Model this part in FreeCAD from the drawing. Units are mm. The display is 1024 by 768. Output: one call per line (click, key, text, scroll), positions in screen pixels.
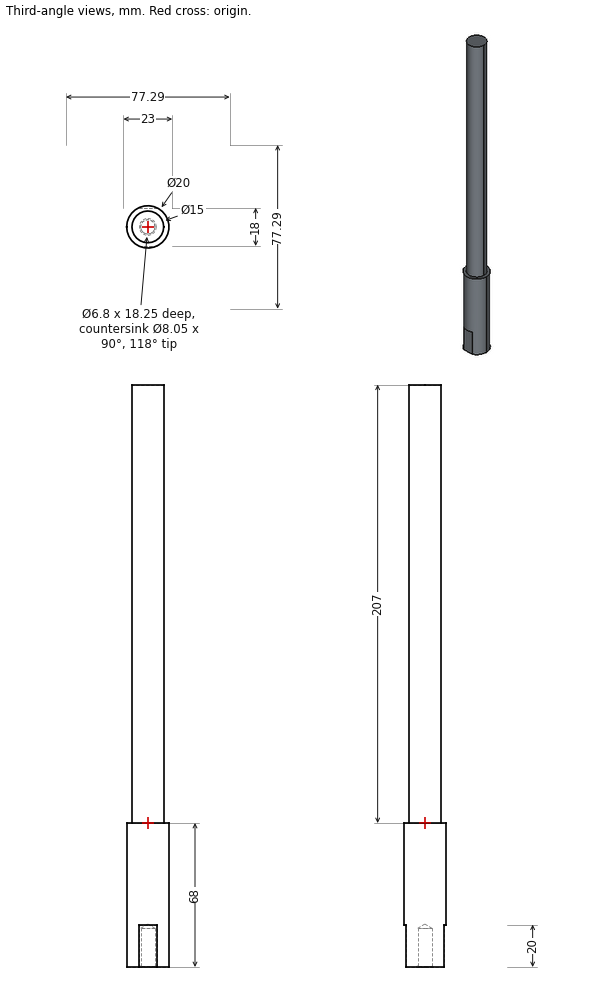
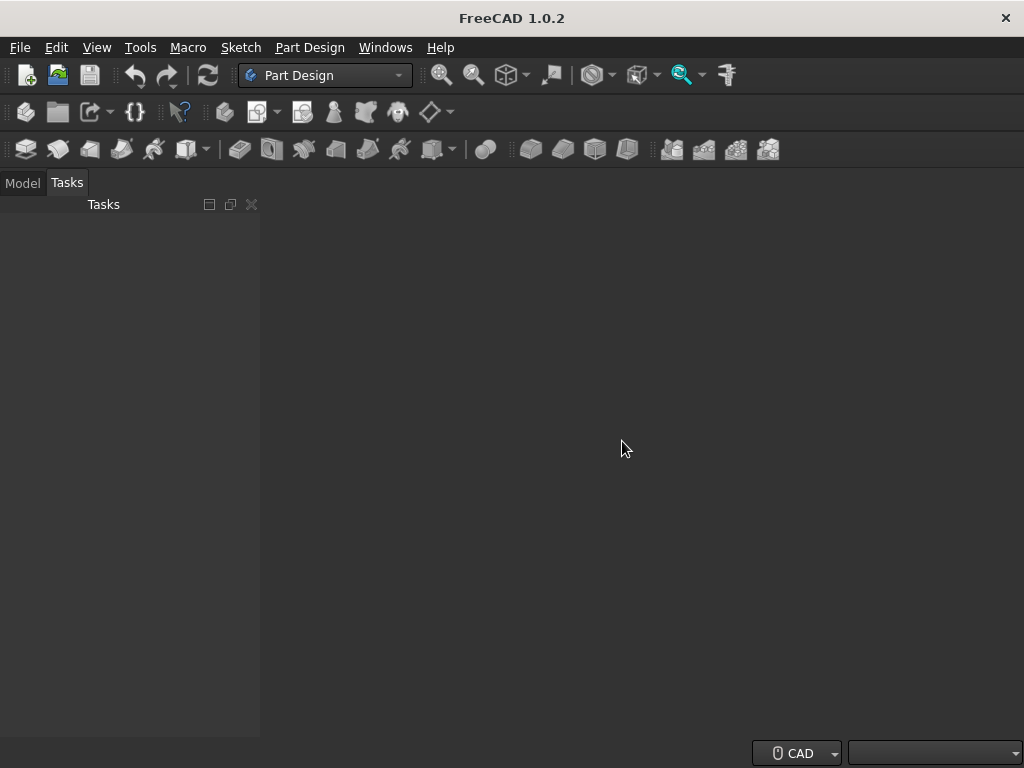
click(26, 76)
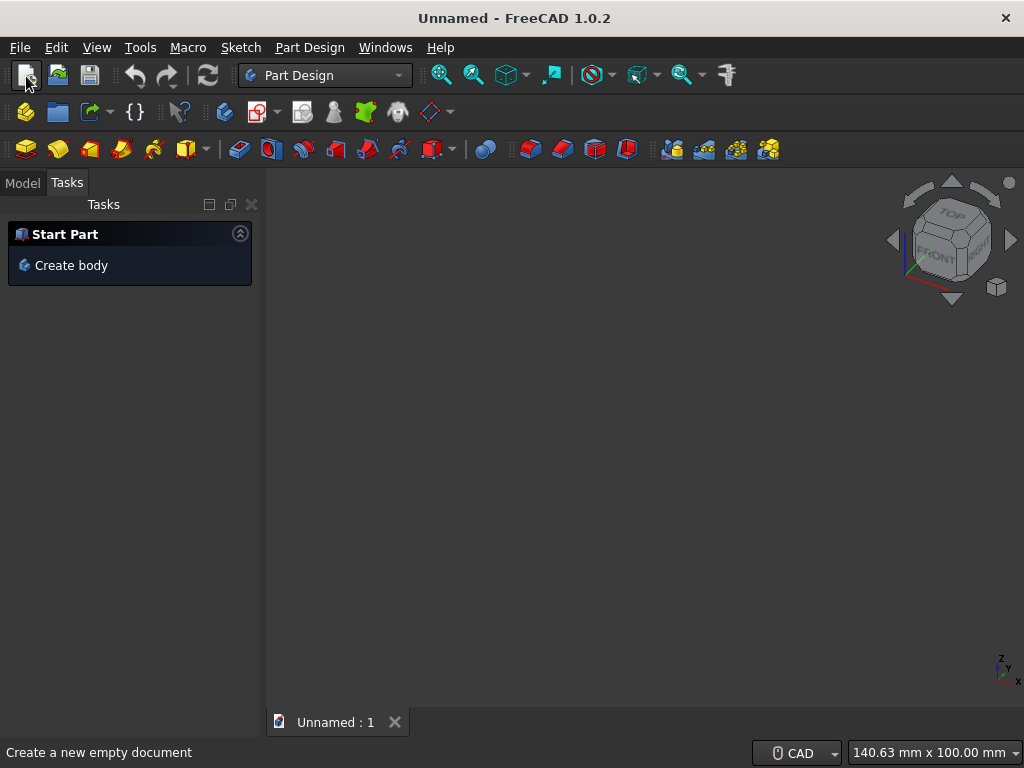
click(258, 112)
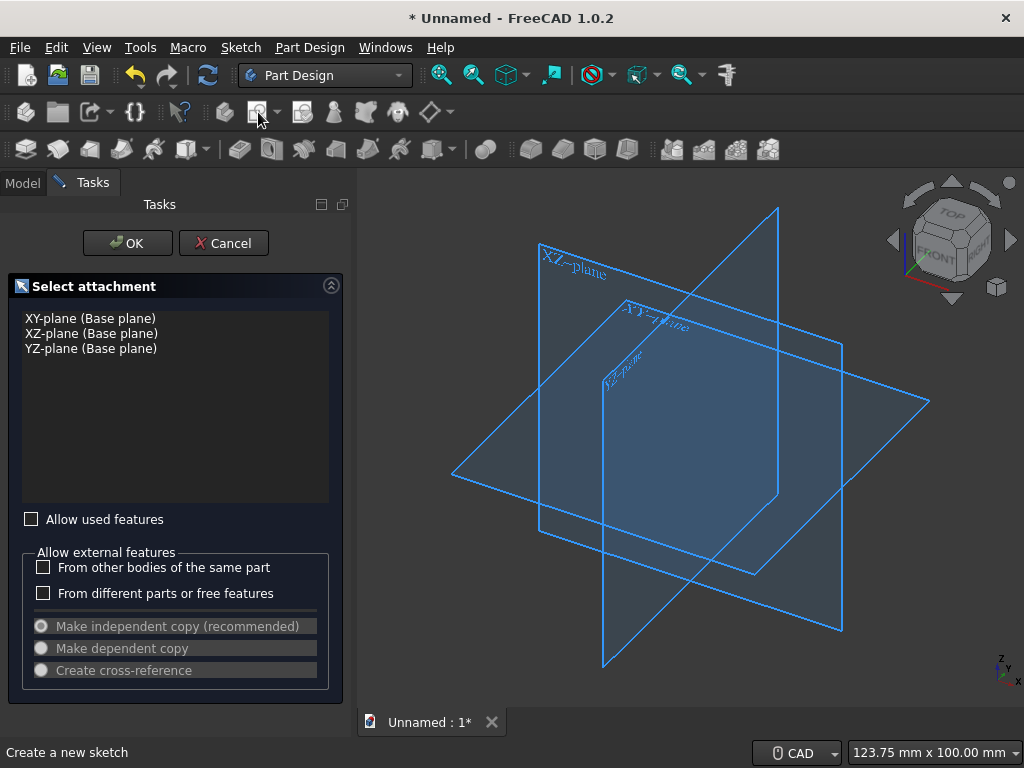
click(82, 318)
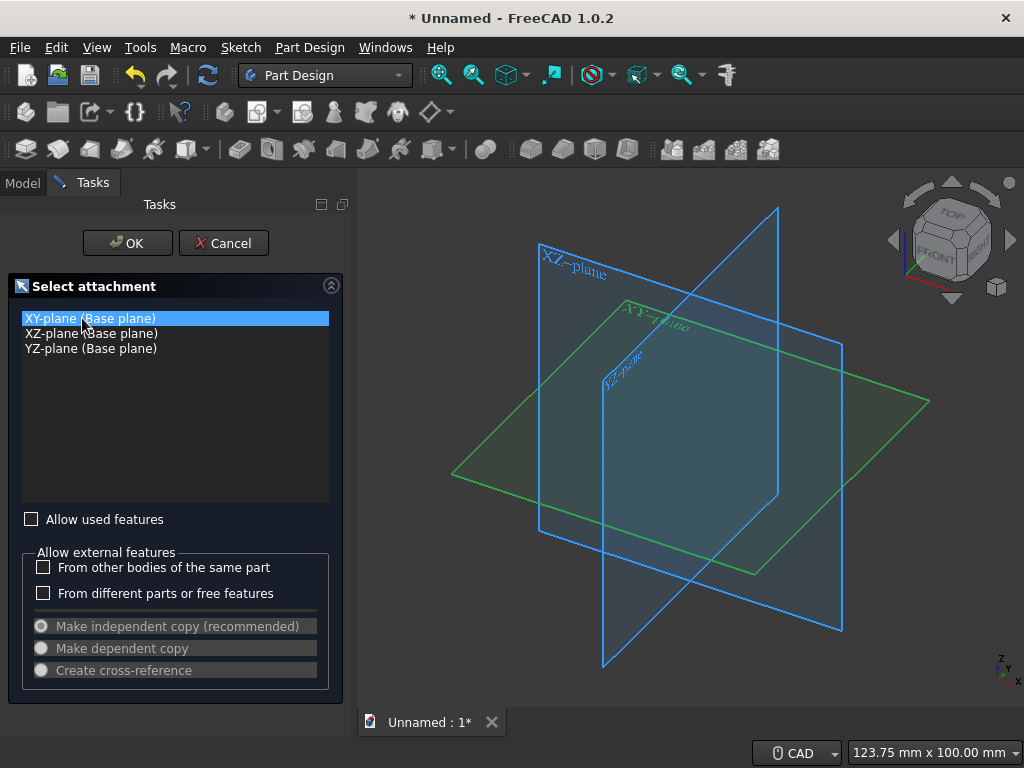
click(128, 243)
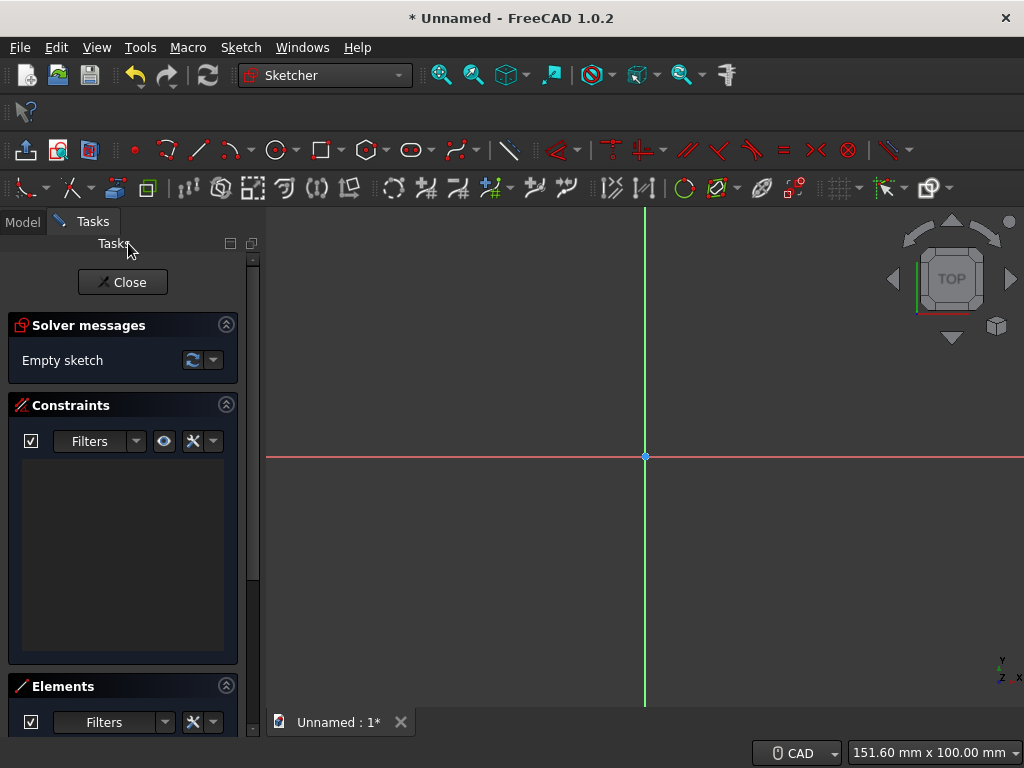
scroll(667, 457, up, 7)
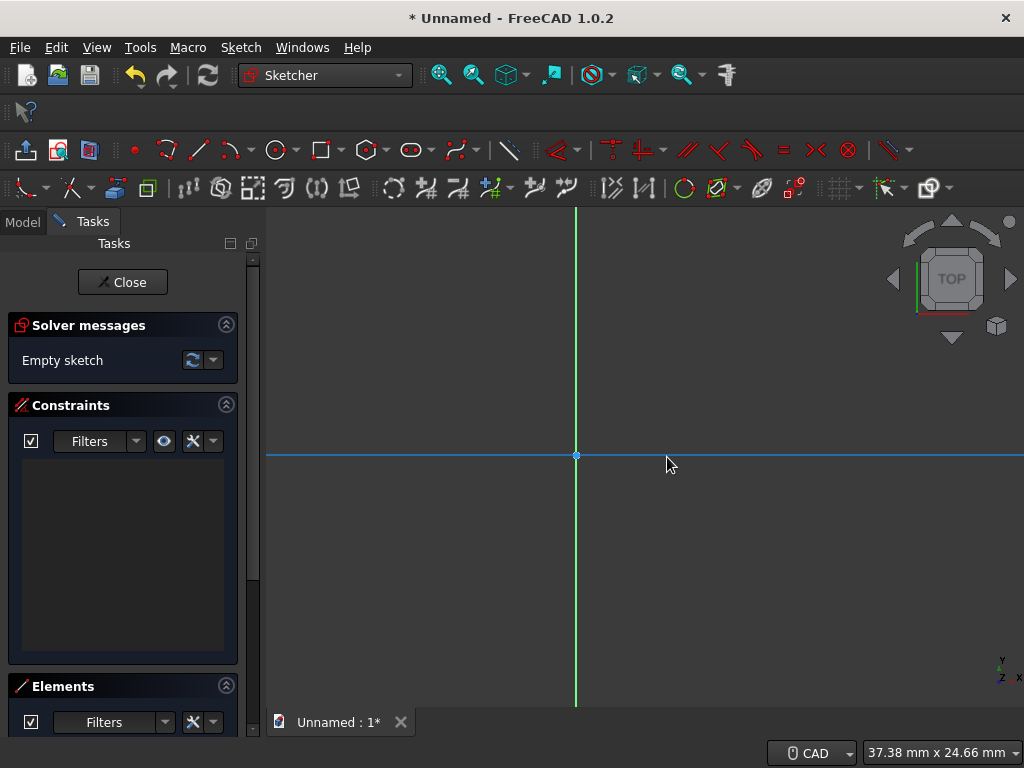
click(276, 150)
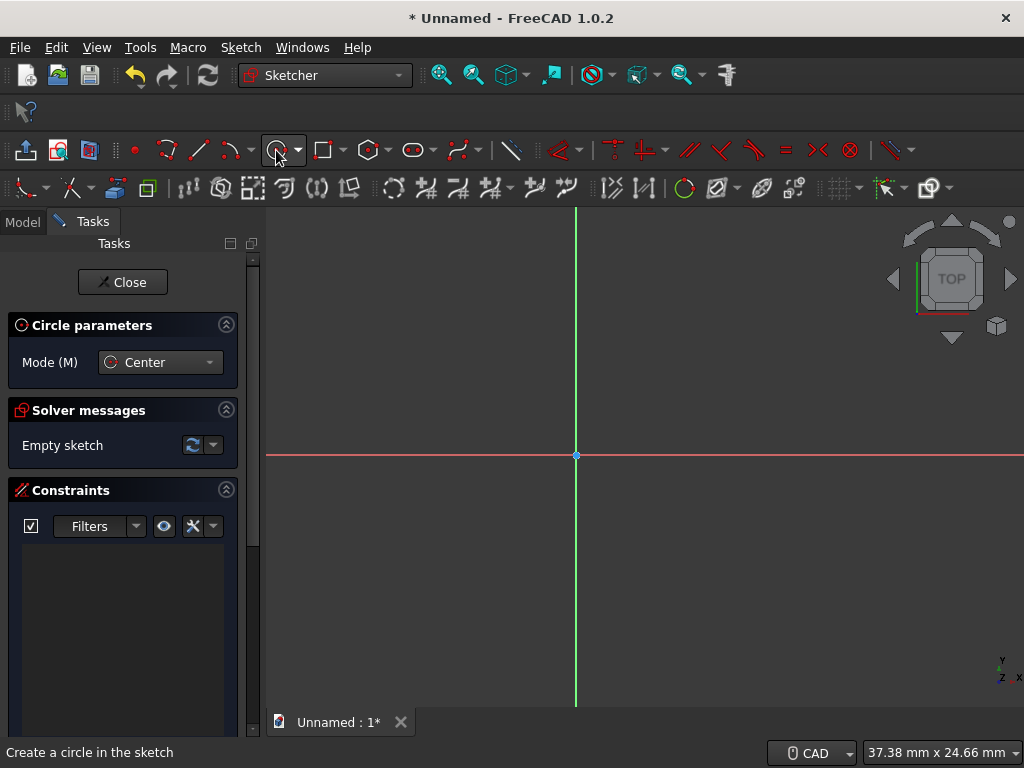
click(576, 455)
click(684, 348)
key(Escape)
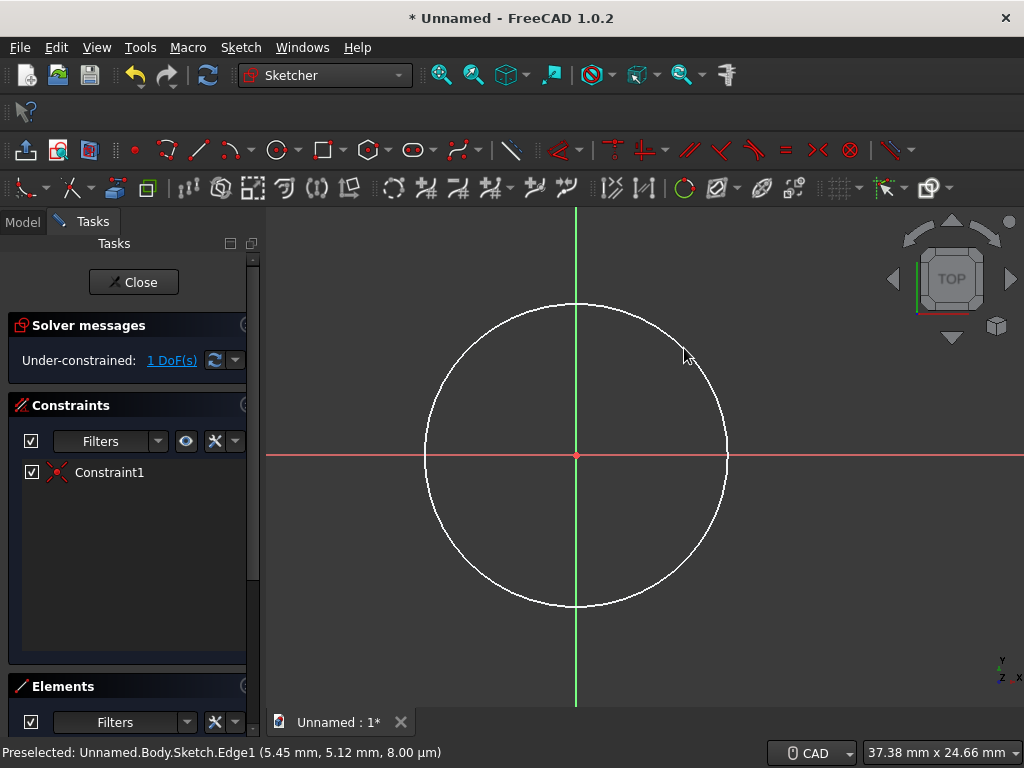
click(683, 348)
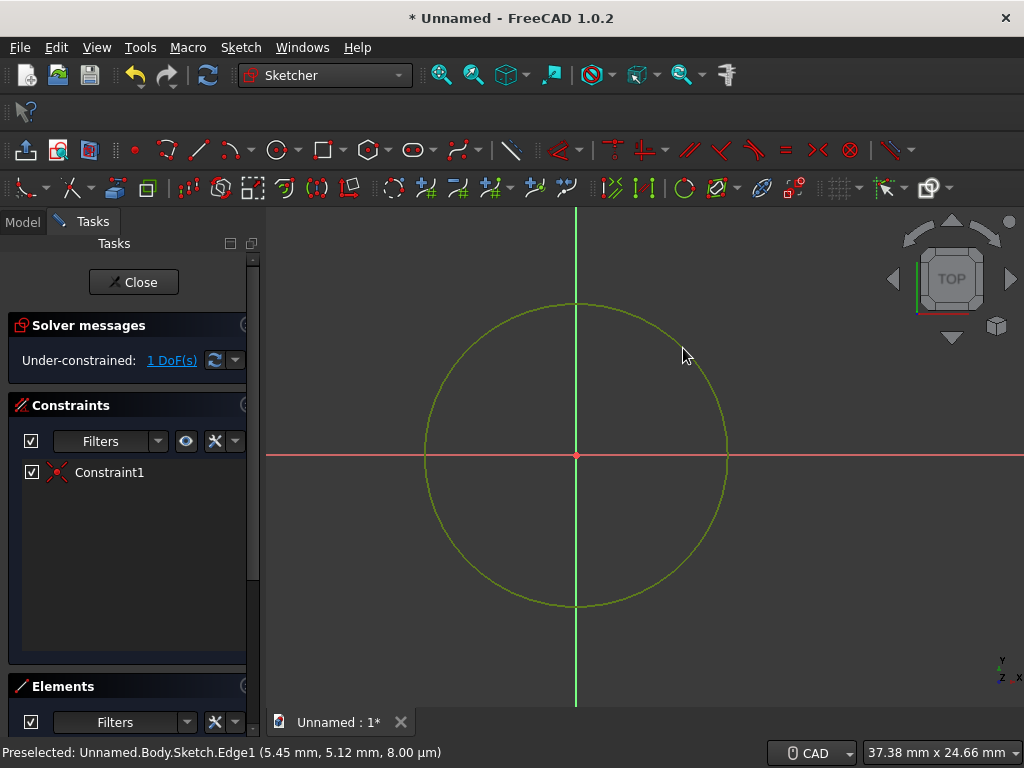
click(582, 150)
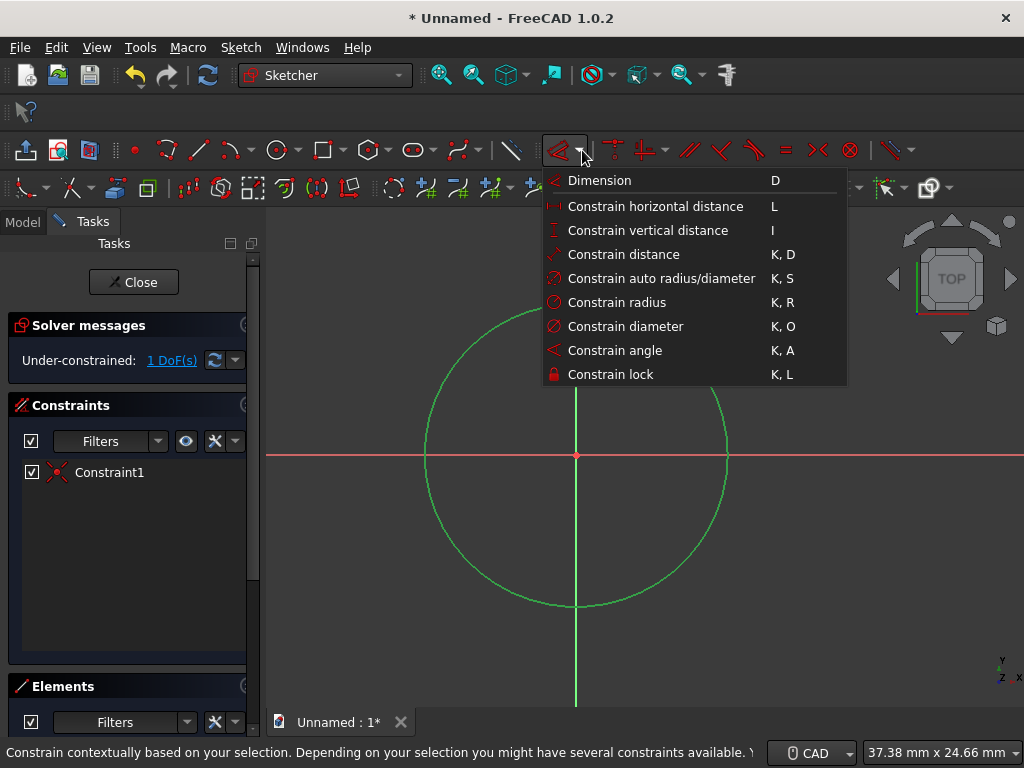
click(695, 326)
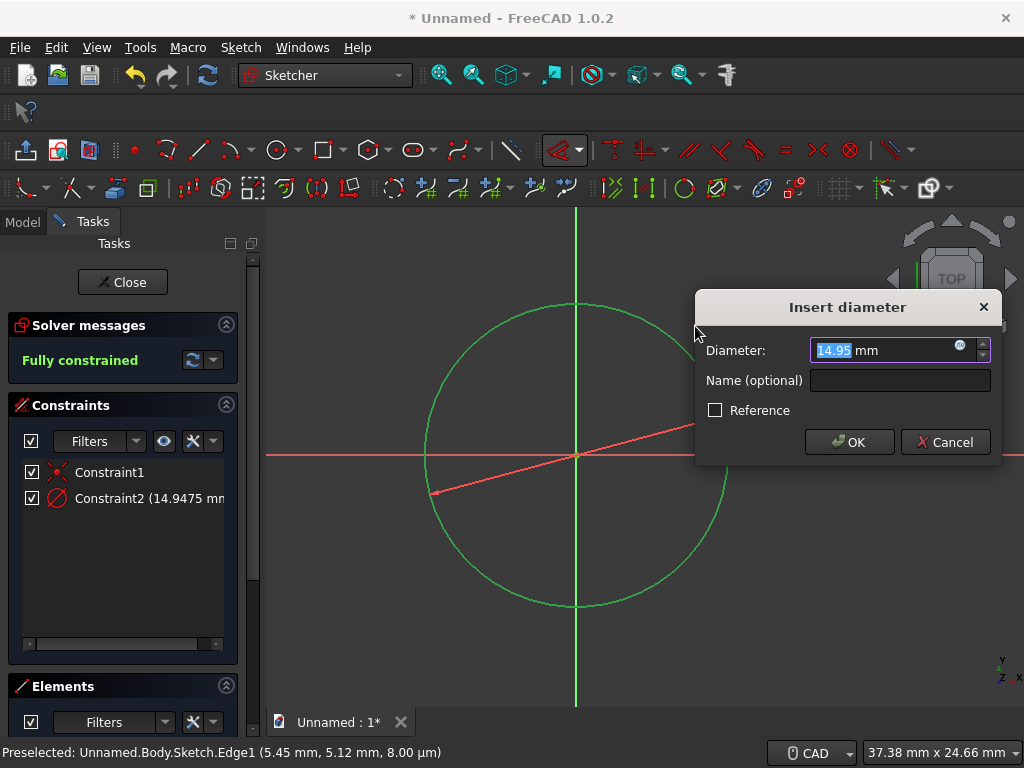
text(15)
key(Return)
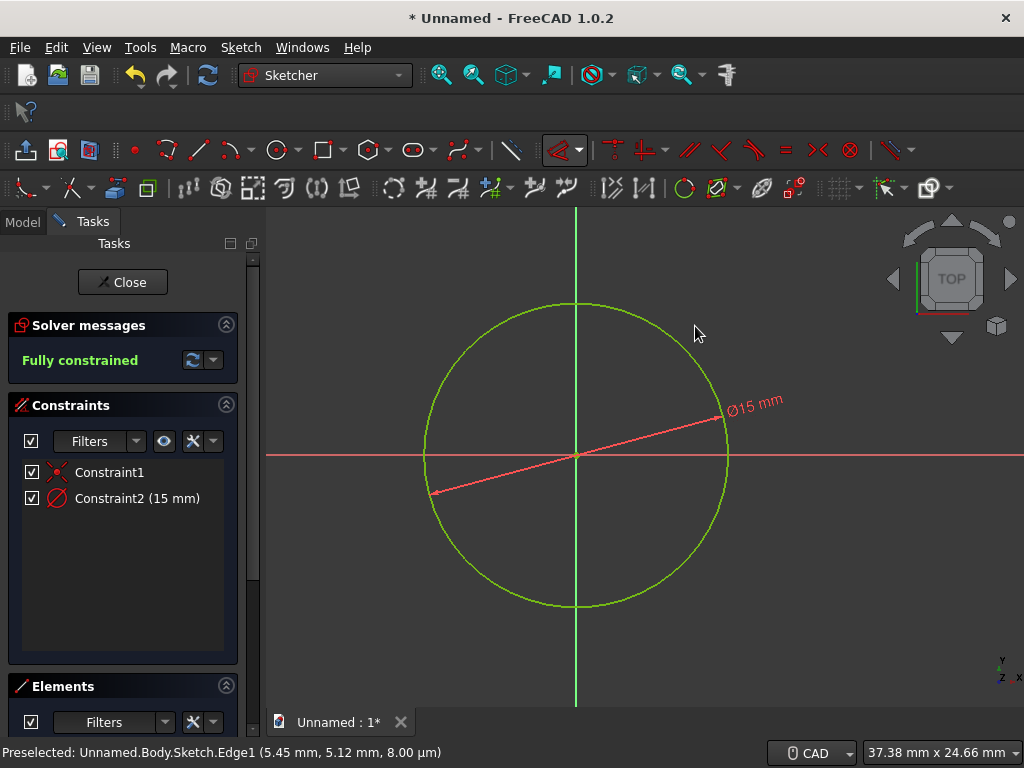
click(123, 282)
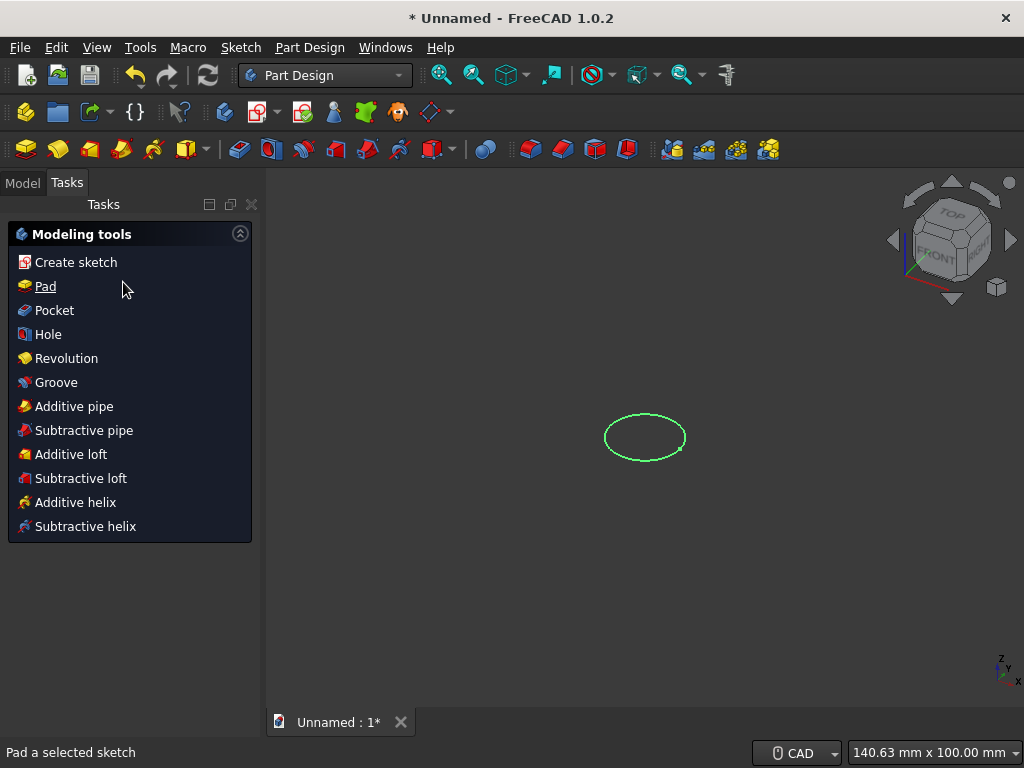
click(26, 150)